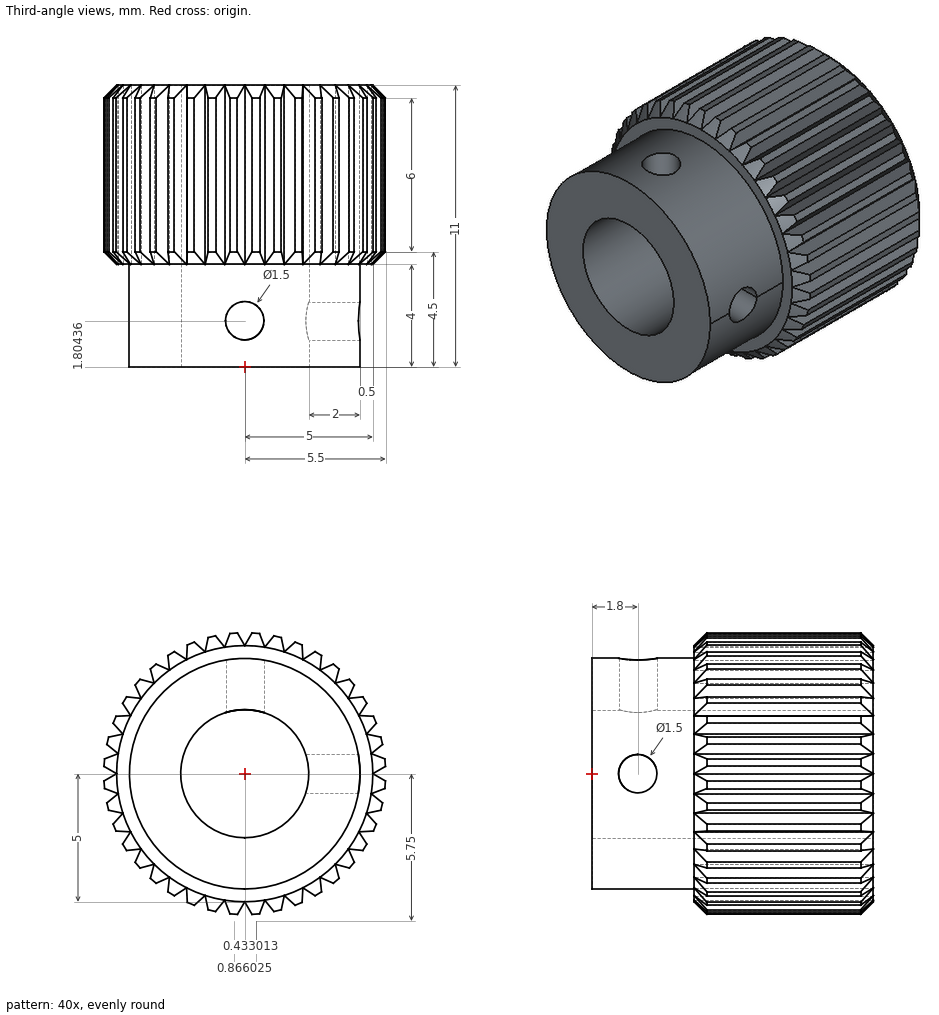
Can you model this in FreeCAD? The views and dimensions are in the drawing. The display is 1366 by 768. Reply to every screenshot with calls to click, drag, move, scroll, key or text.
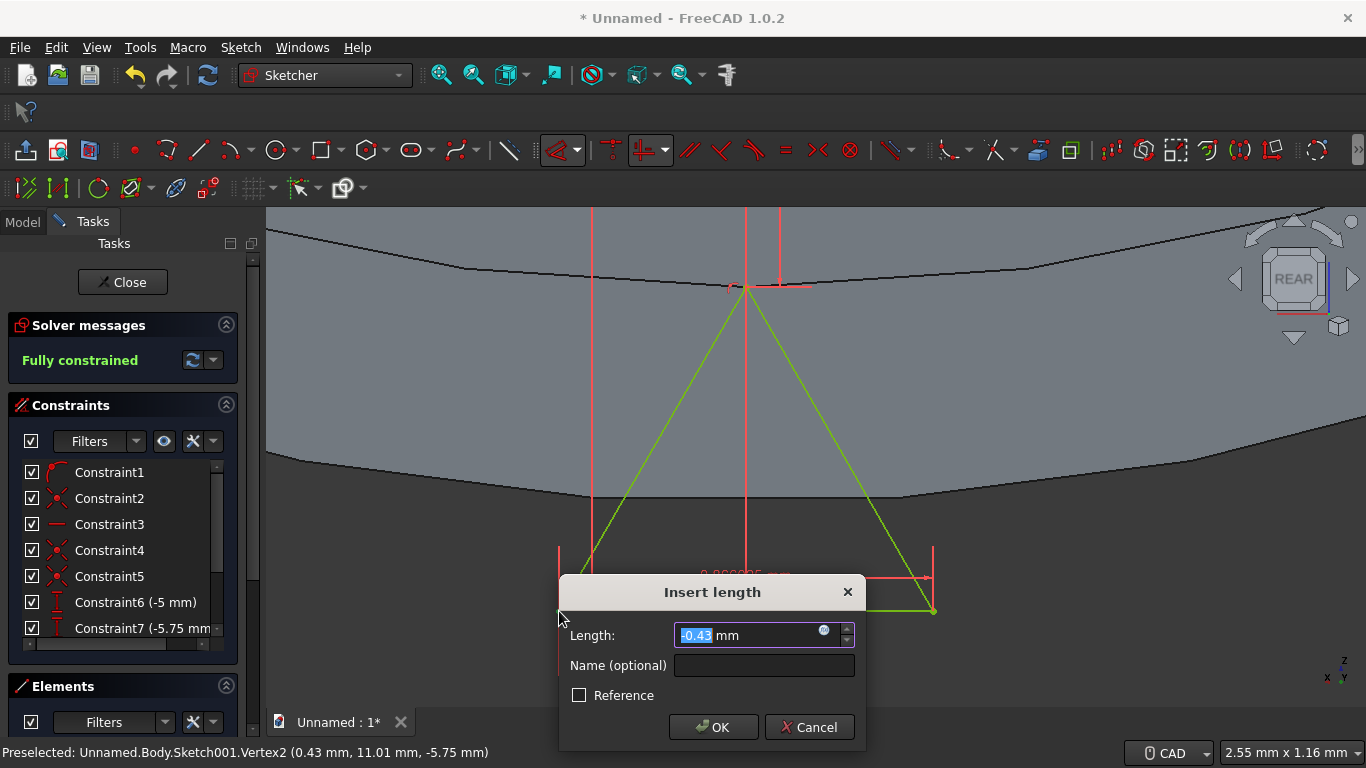
text(-0.433013)
key(Return)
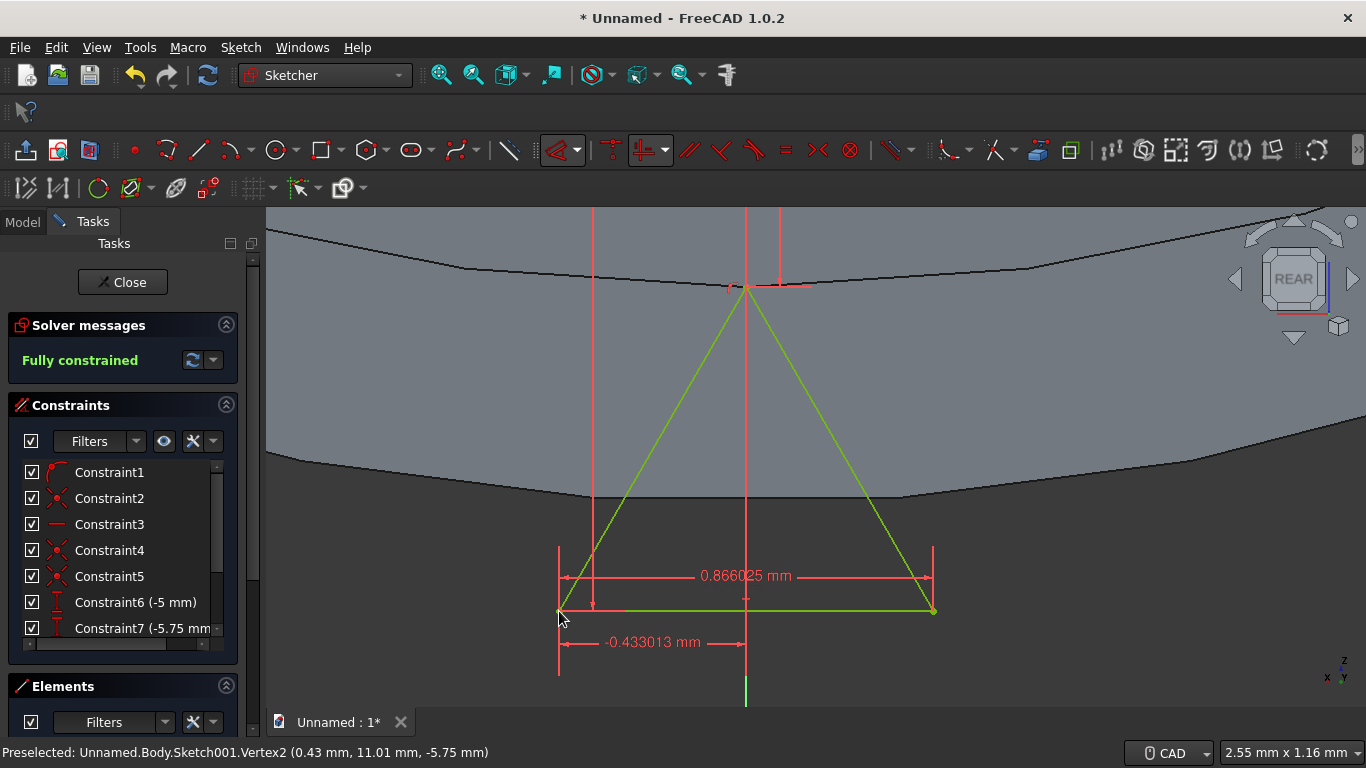
click(123, 282)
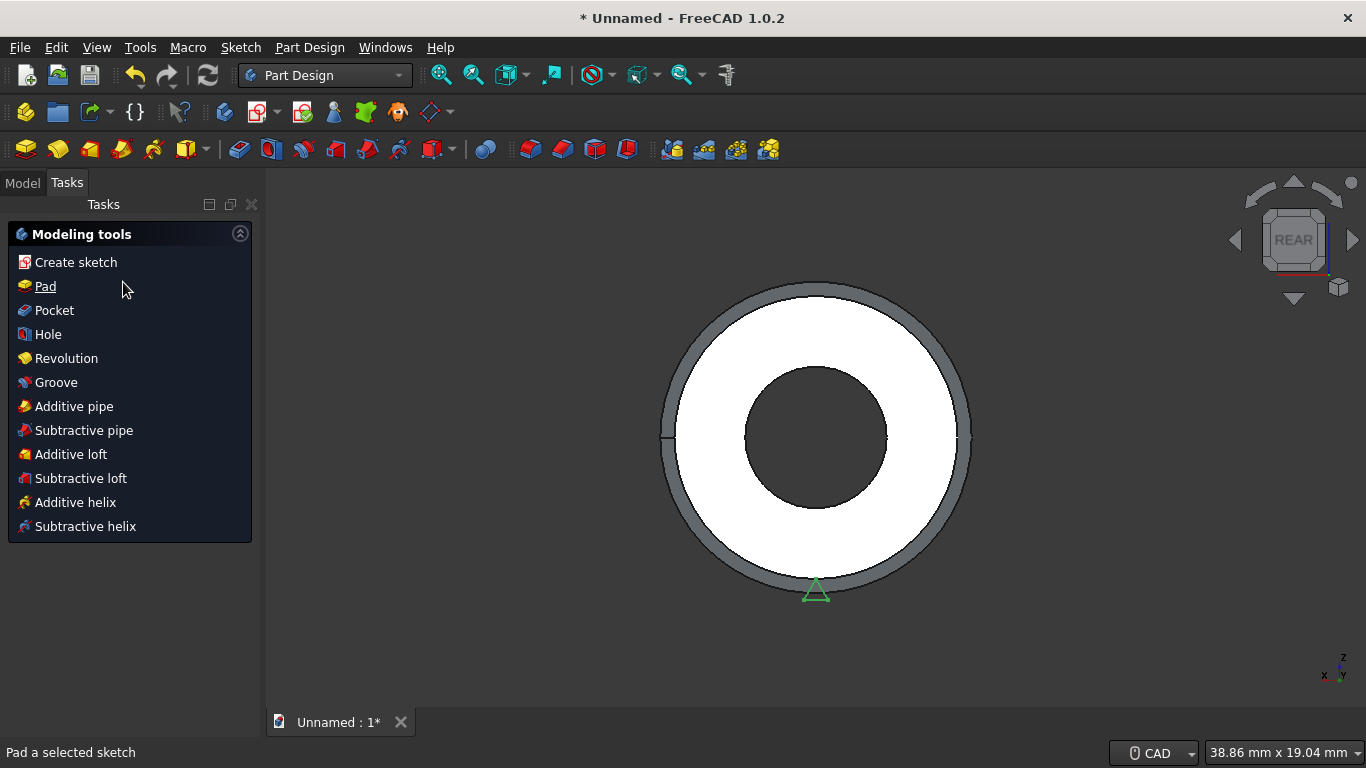
click(240, 150)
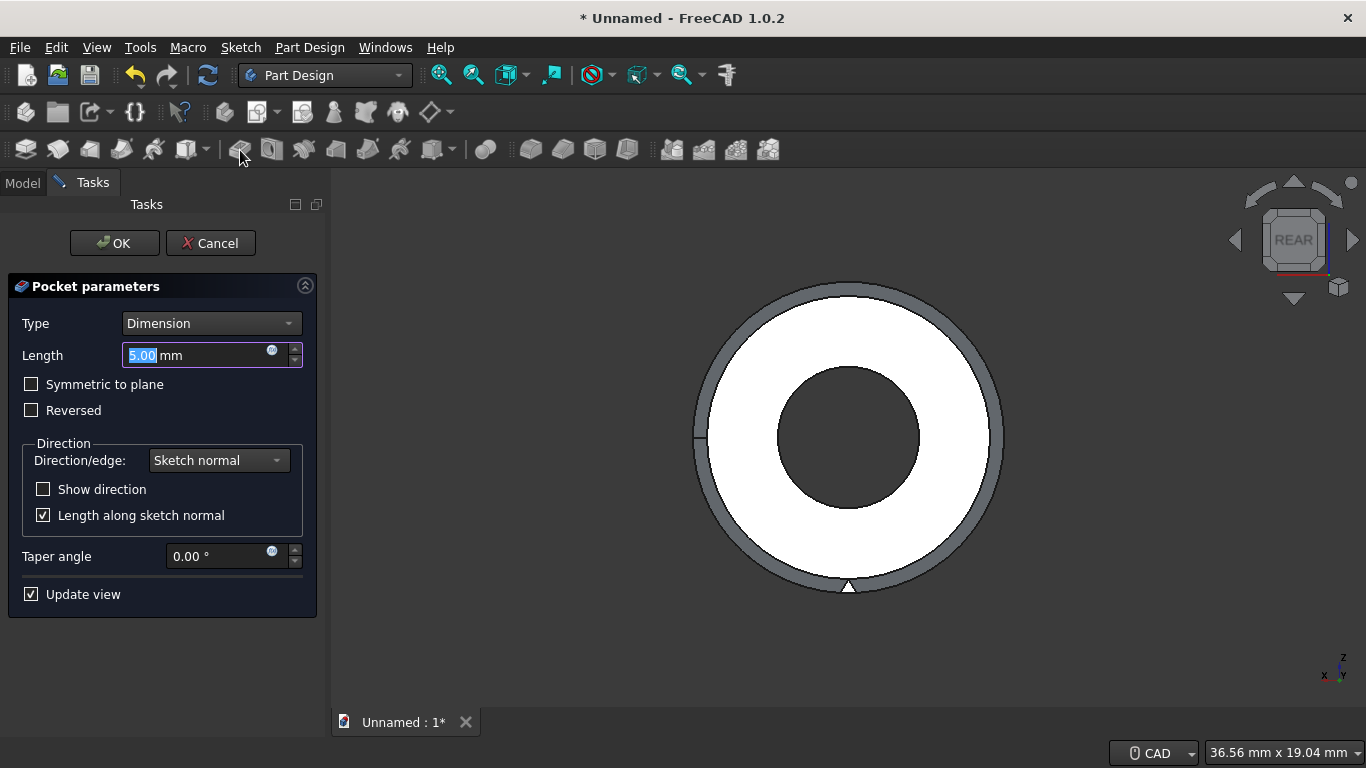
click(212, 324)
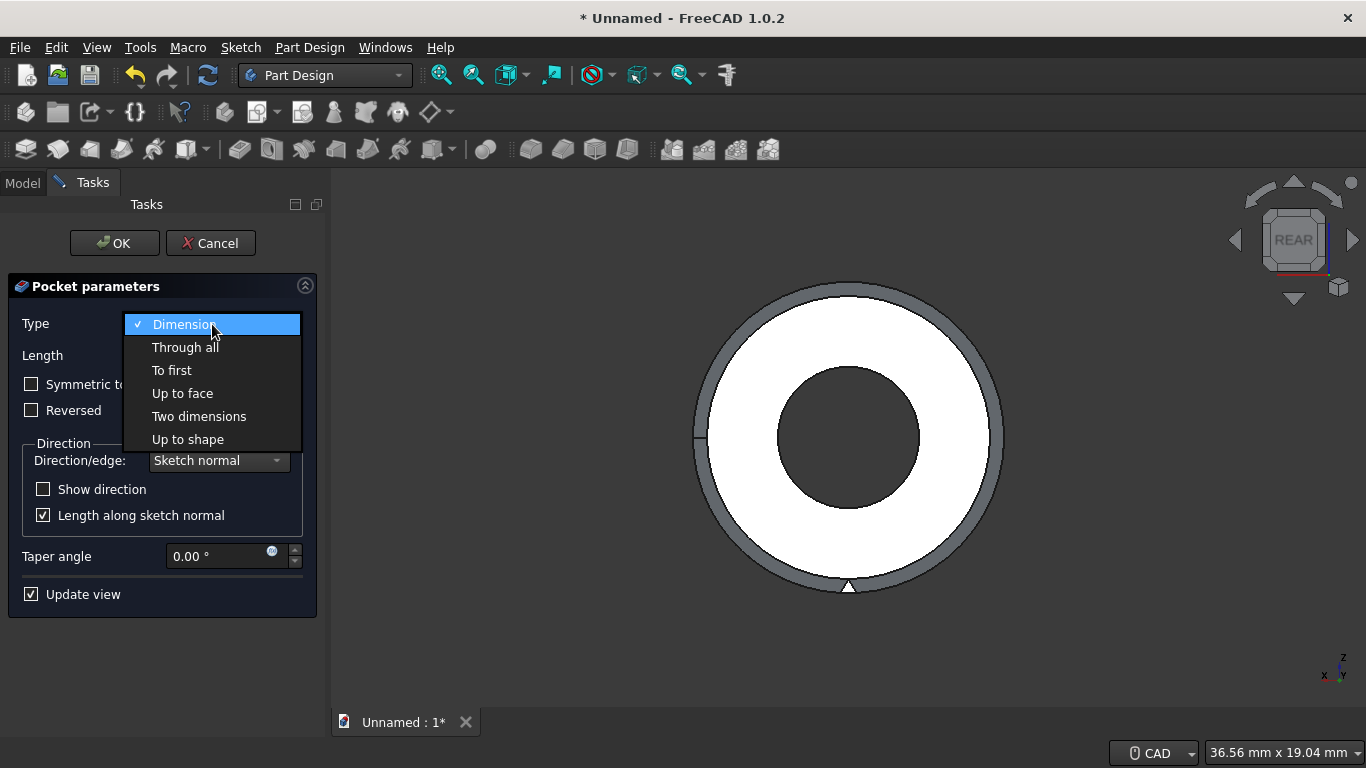
click(212, 348)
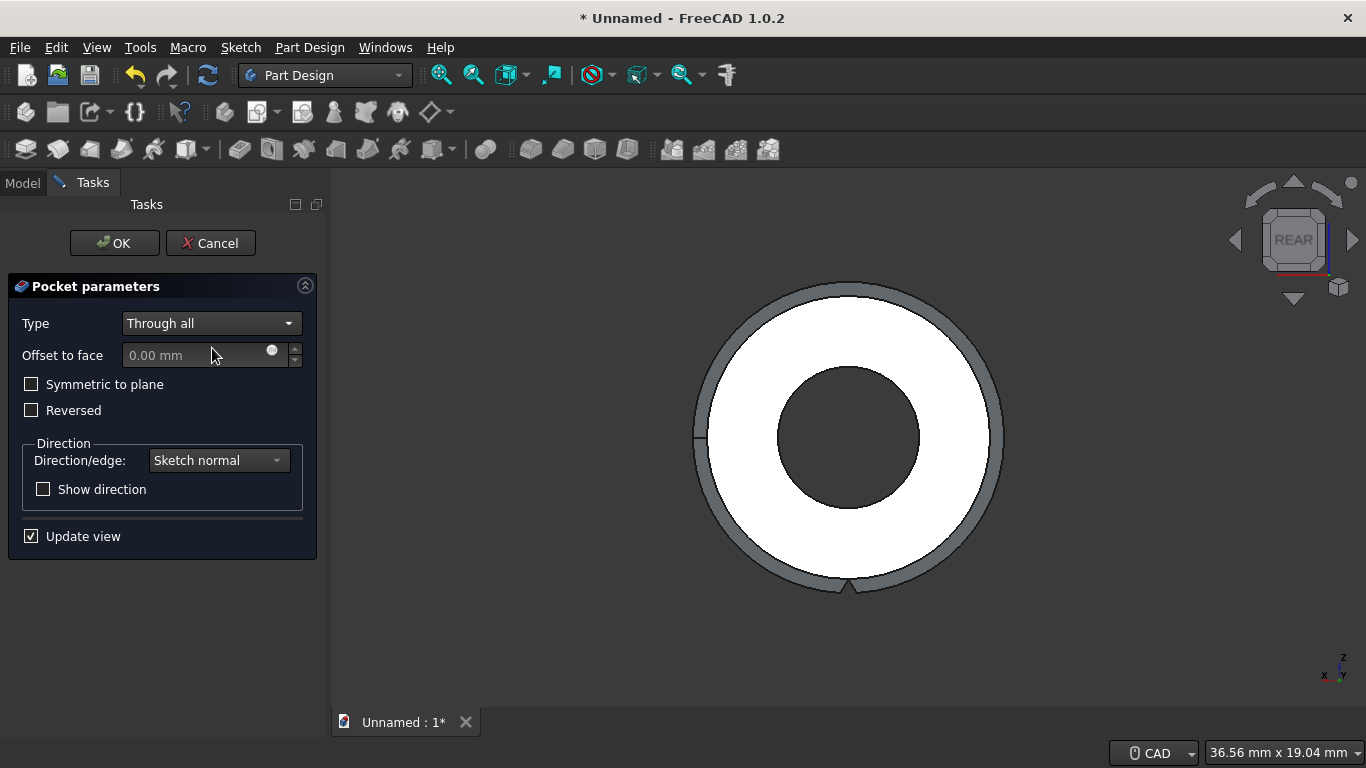
click(115, 243)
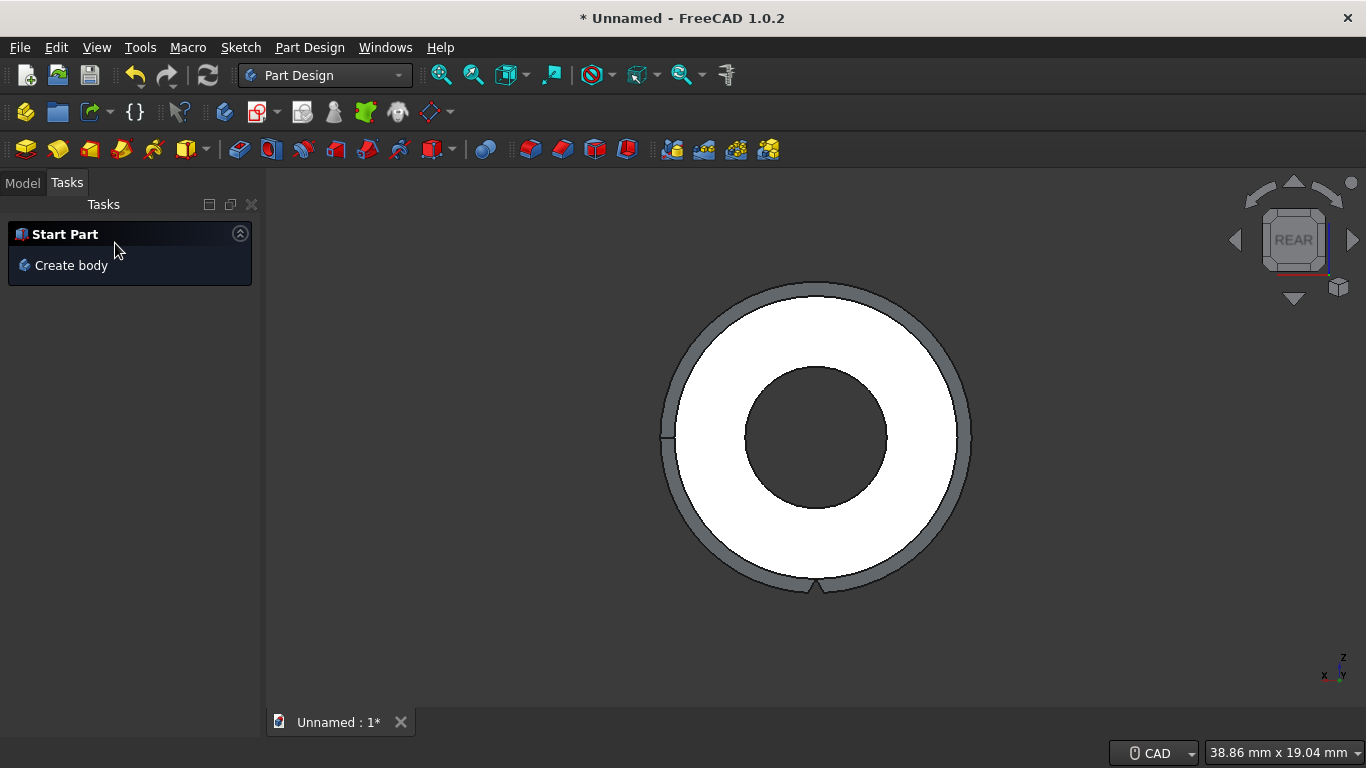
click(23, 182)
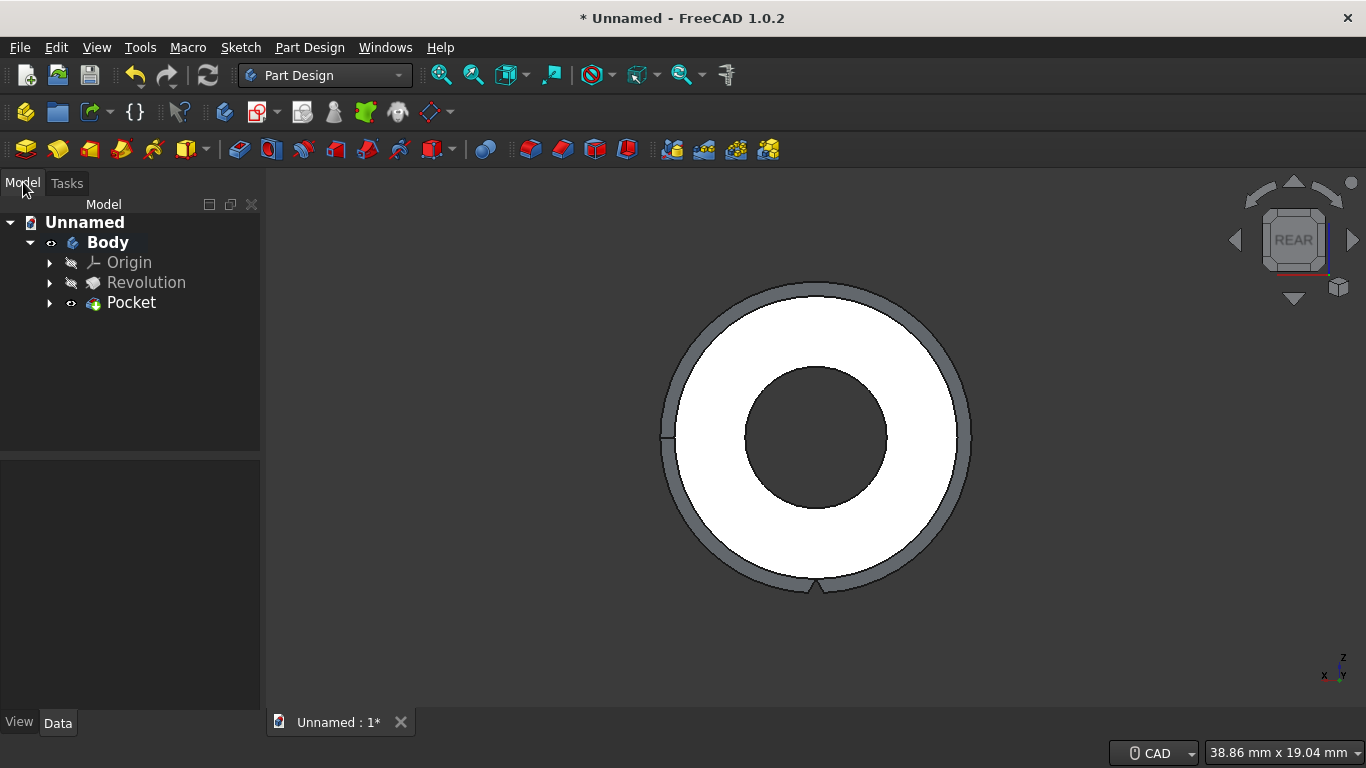
click(116, 303)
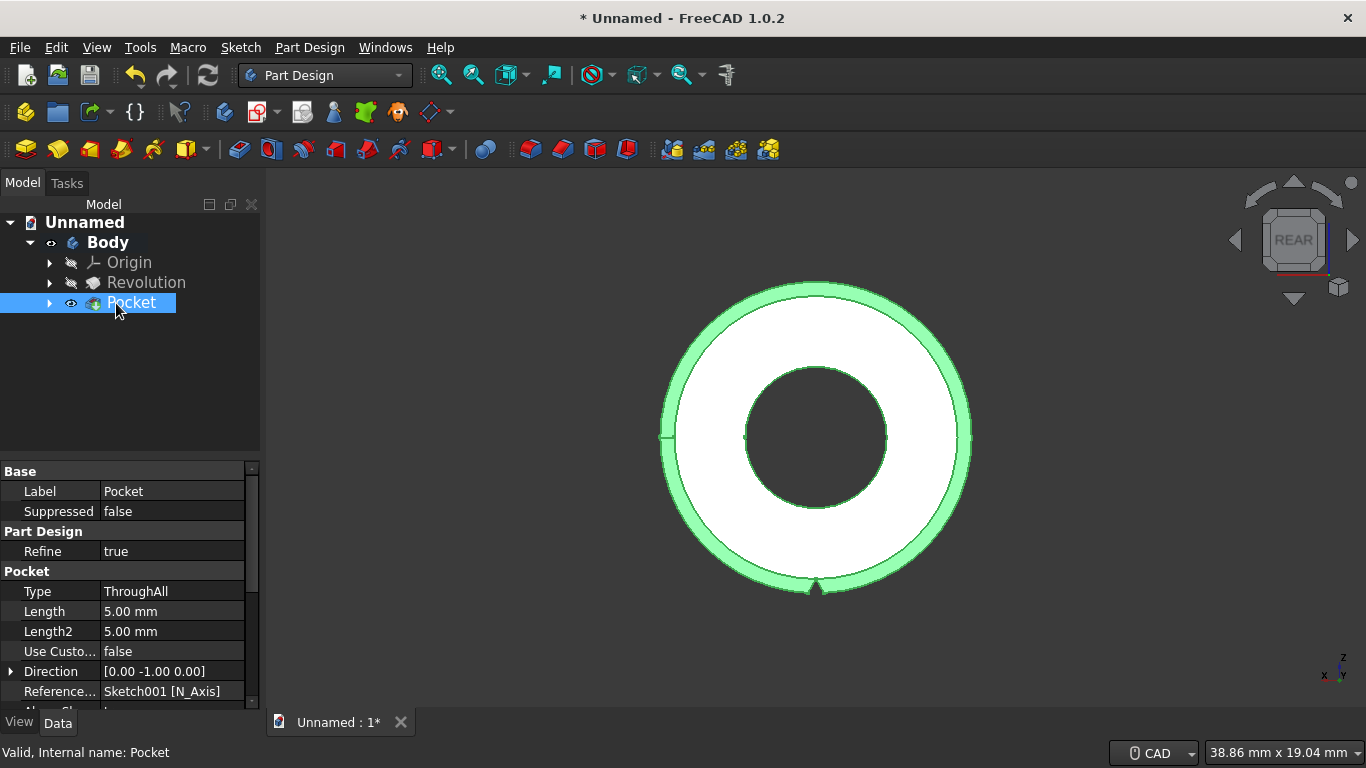
click(736, 150)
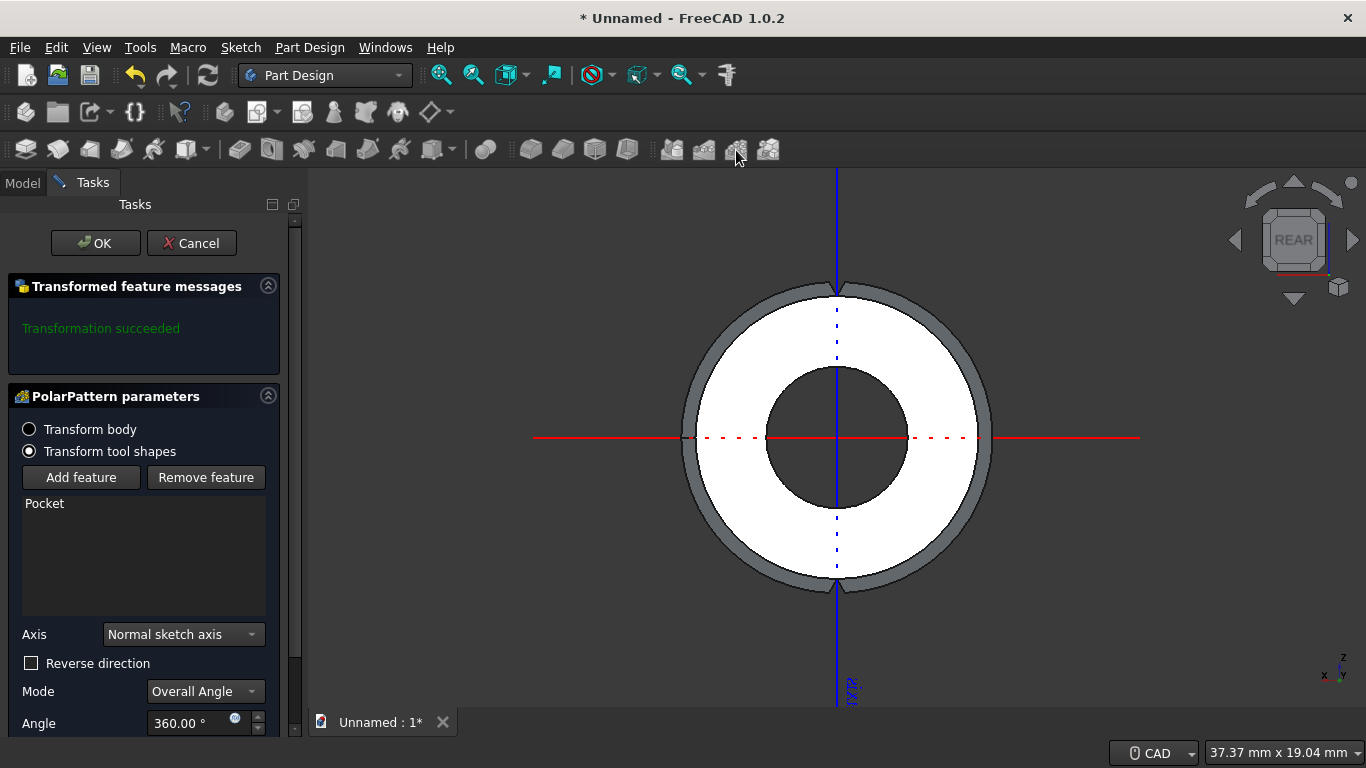
click(184, 634)